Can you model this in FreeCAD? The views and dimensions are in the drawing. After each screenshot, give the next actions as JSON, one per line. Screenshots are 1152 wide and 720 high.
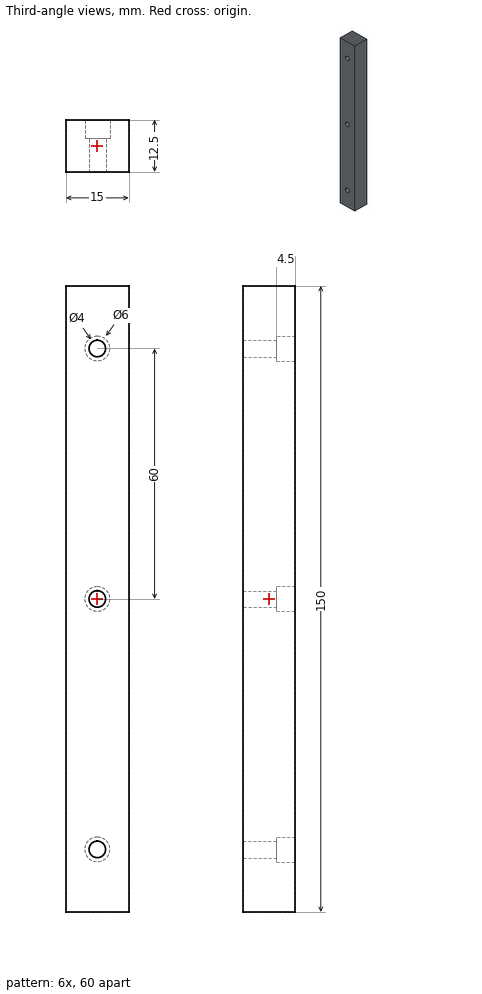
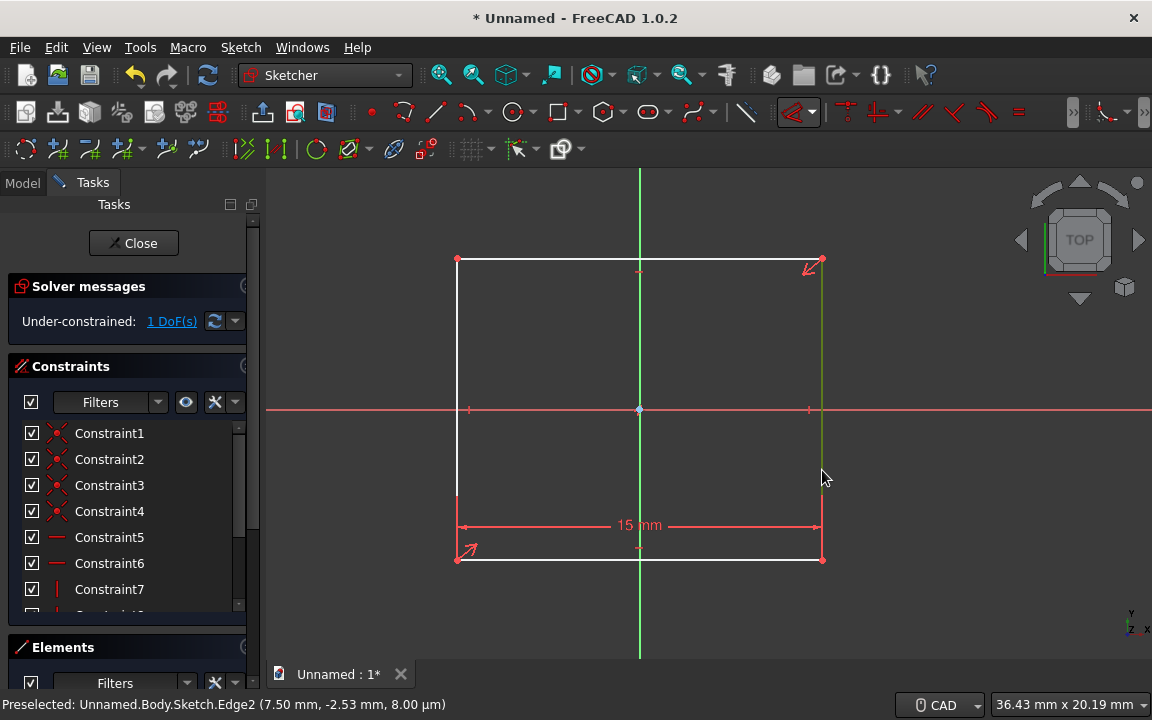
{"action": "key", "text": "i"}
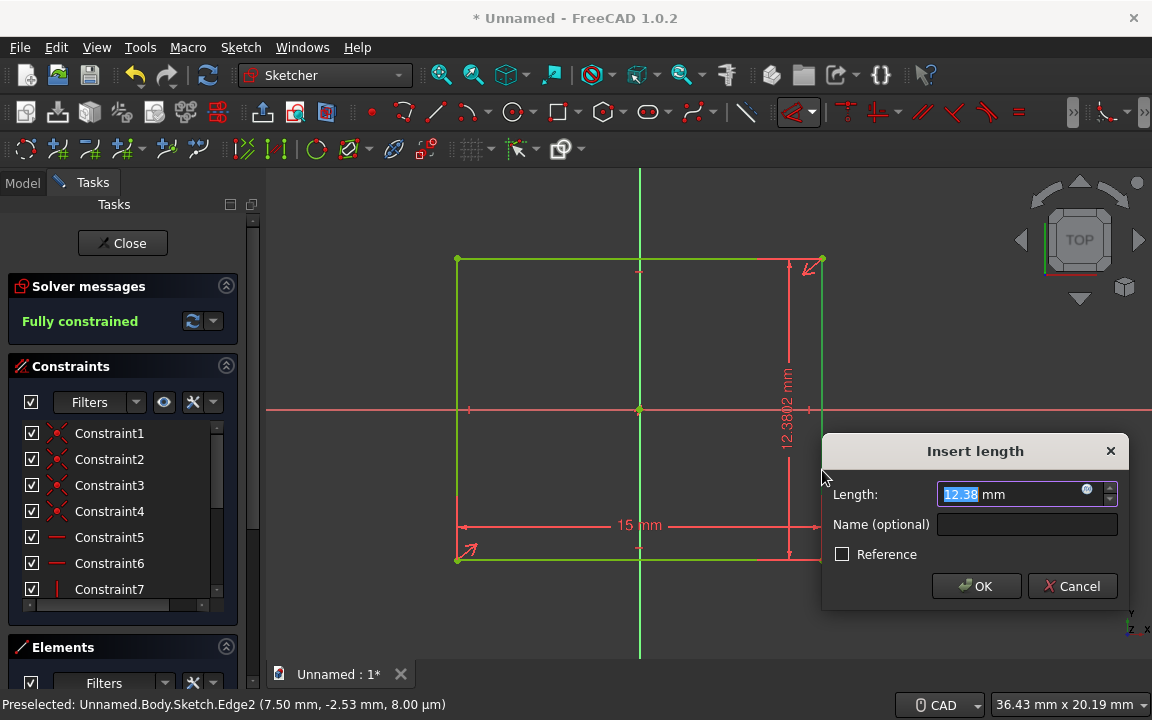
{"action": "type", "text": "12.5"}
{"action": "key", "text": "Return"}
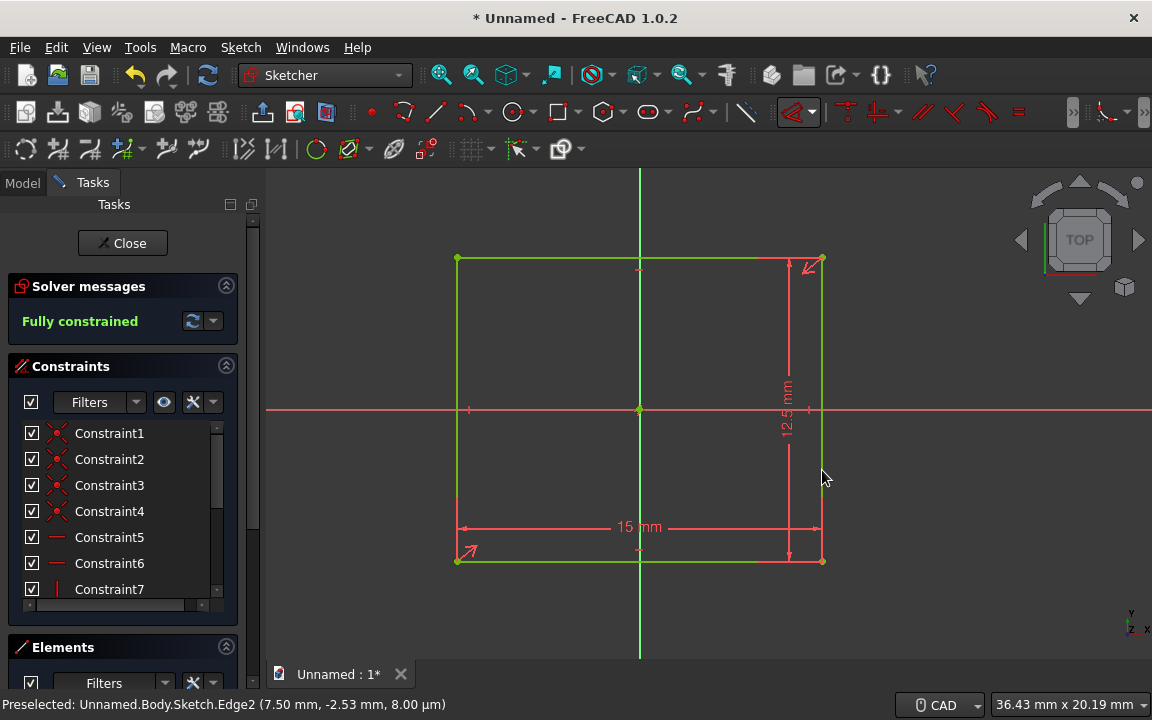
{"action": "left_click", "coordinate": [123, 243]}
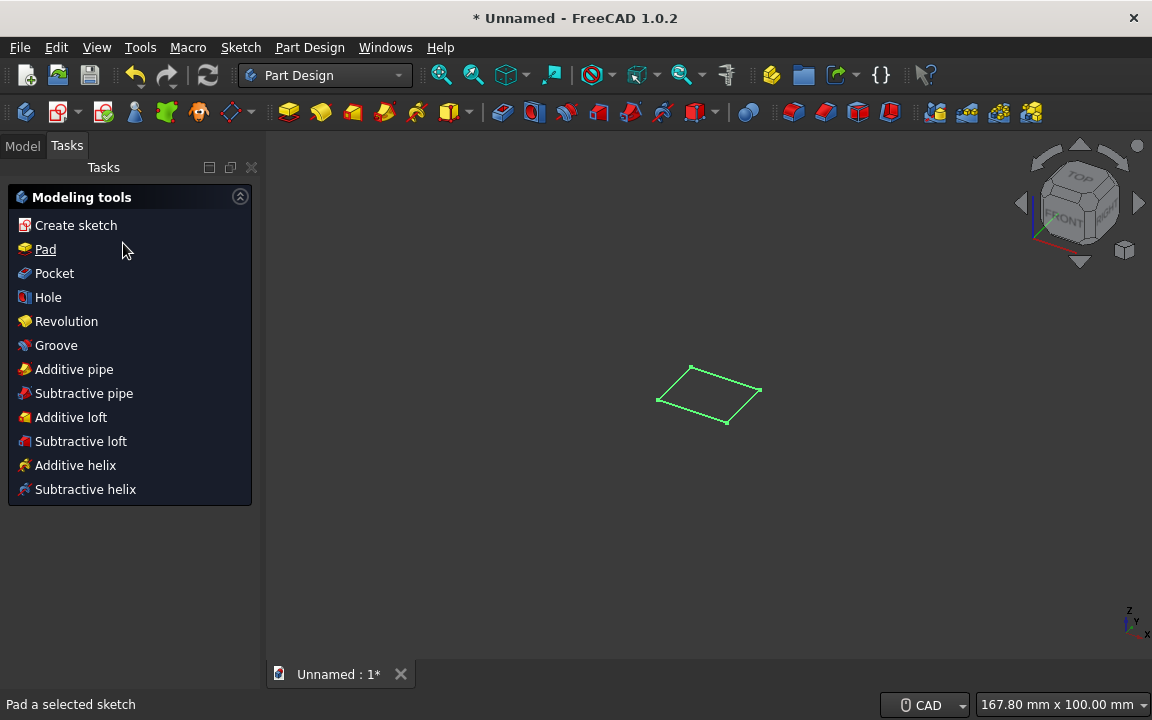
{"action": "left_click", "coordinate": [290, 112]}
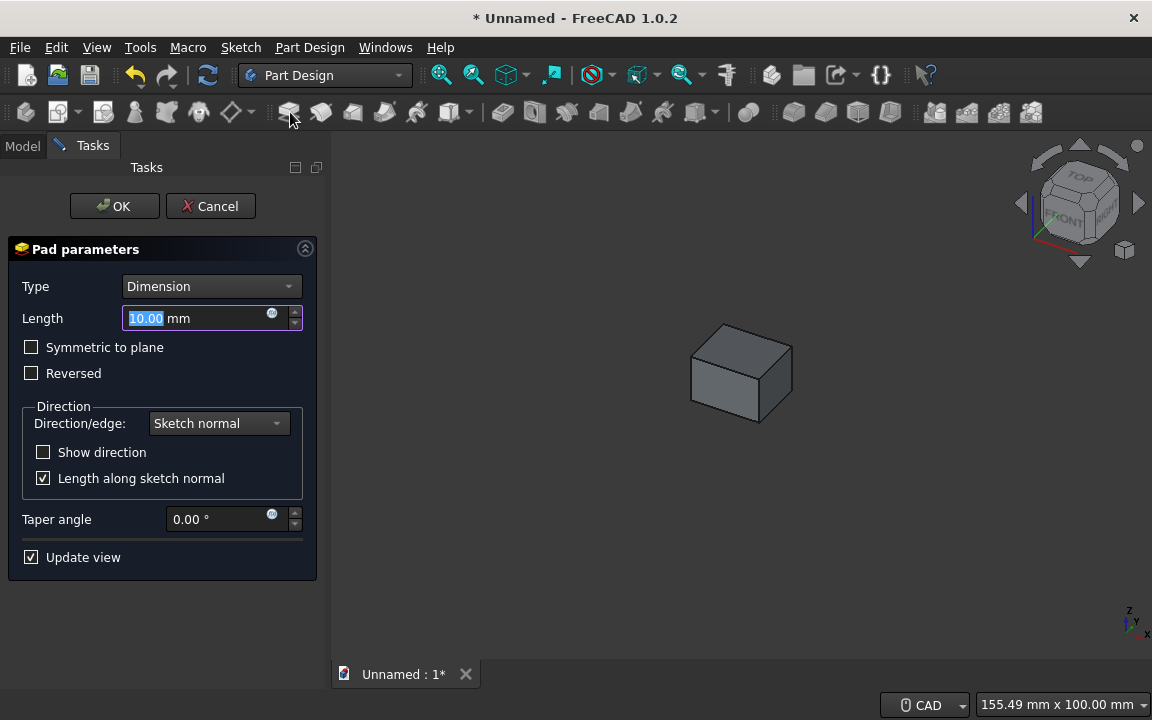
{"action": "type", "text": "150"}
{"action": "key", "text": "Tab"}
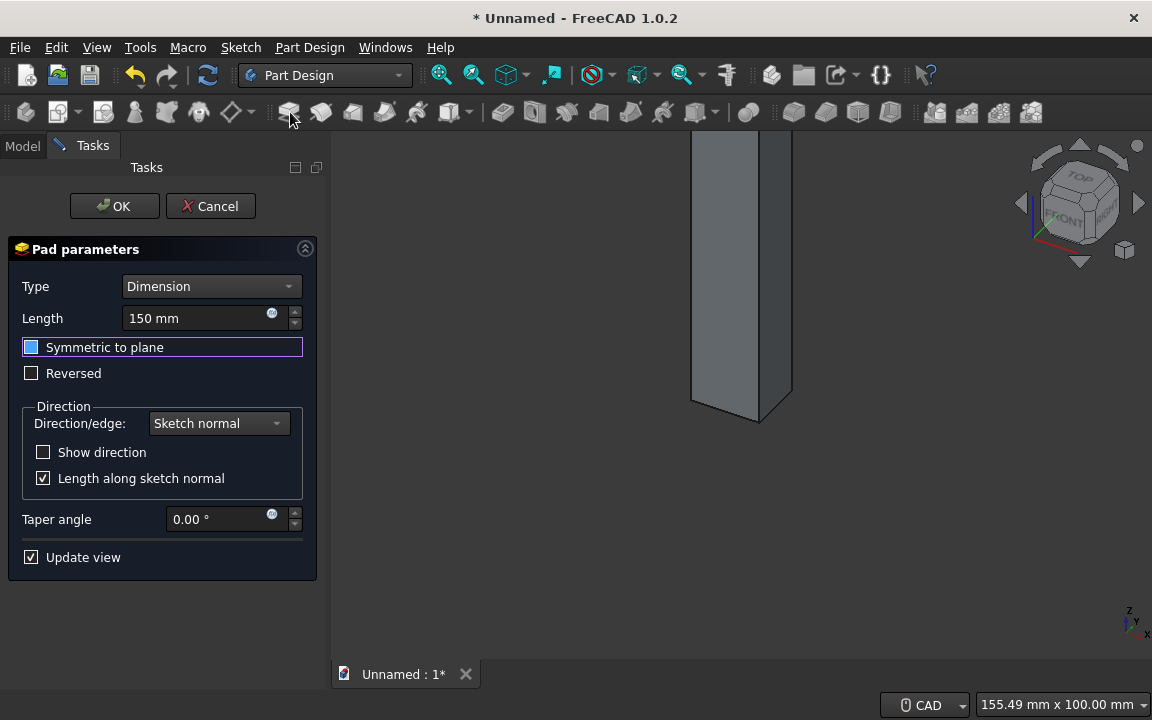
{"action": "left_click", "coordinate": [30, 347]}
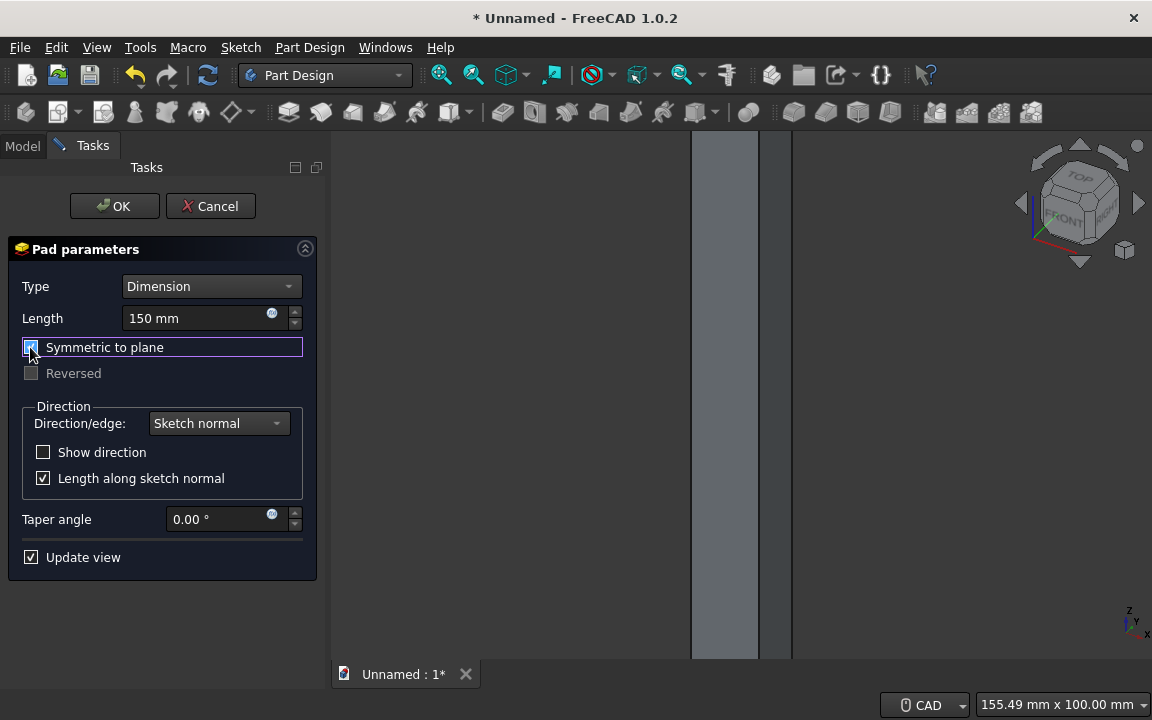
{"action": "left_click", "coordinate": [115, 206]}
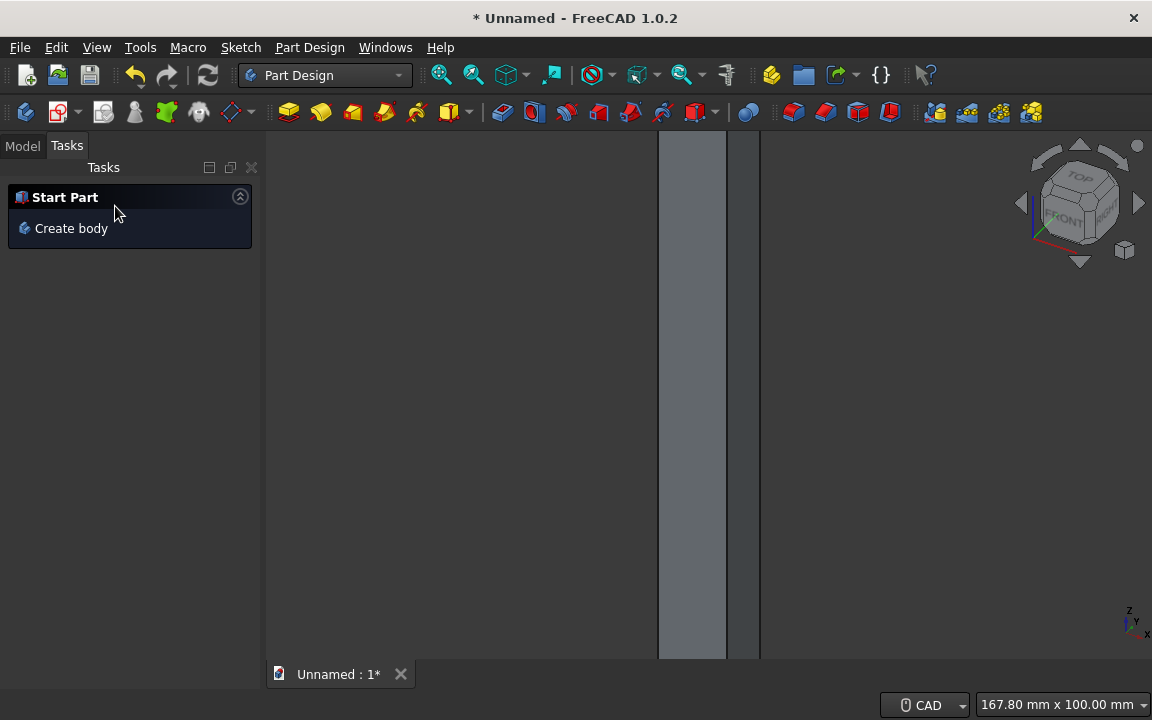
{"action": "key", "text": "v f"}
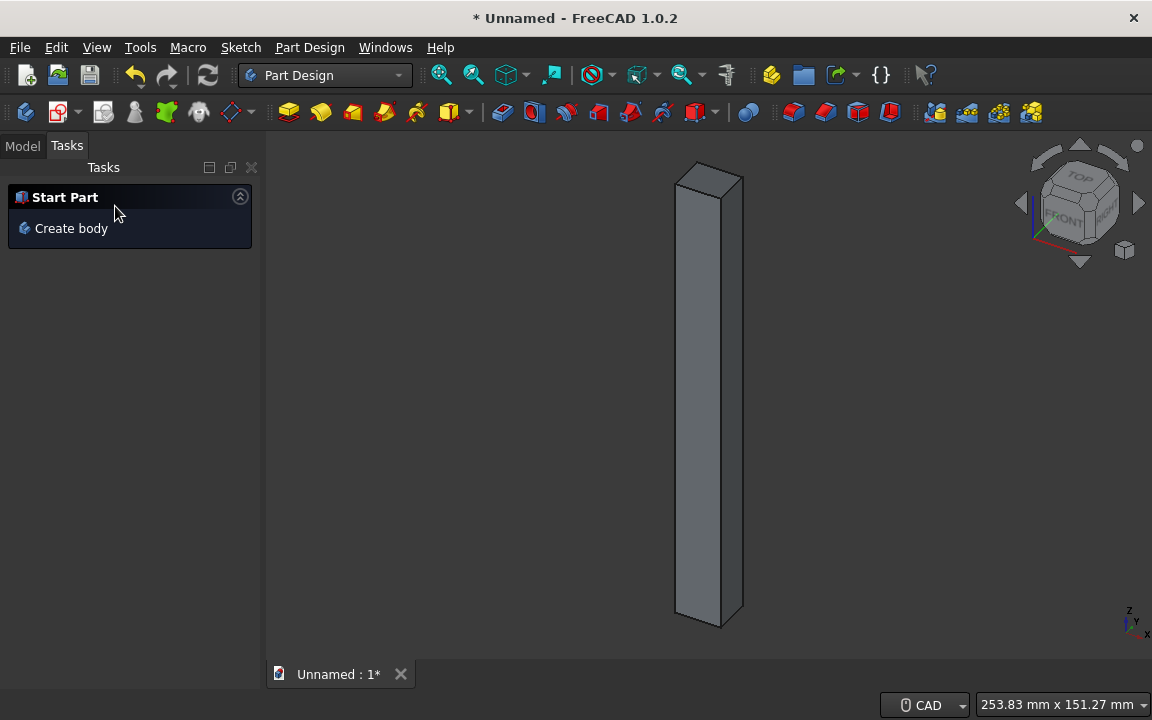
{"action": "key", "text": "4"}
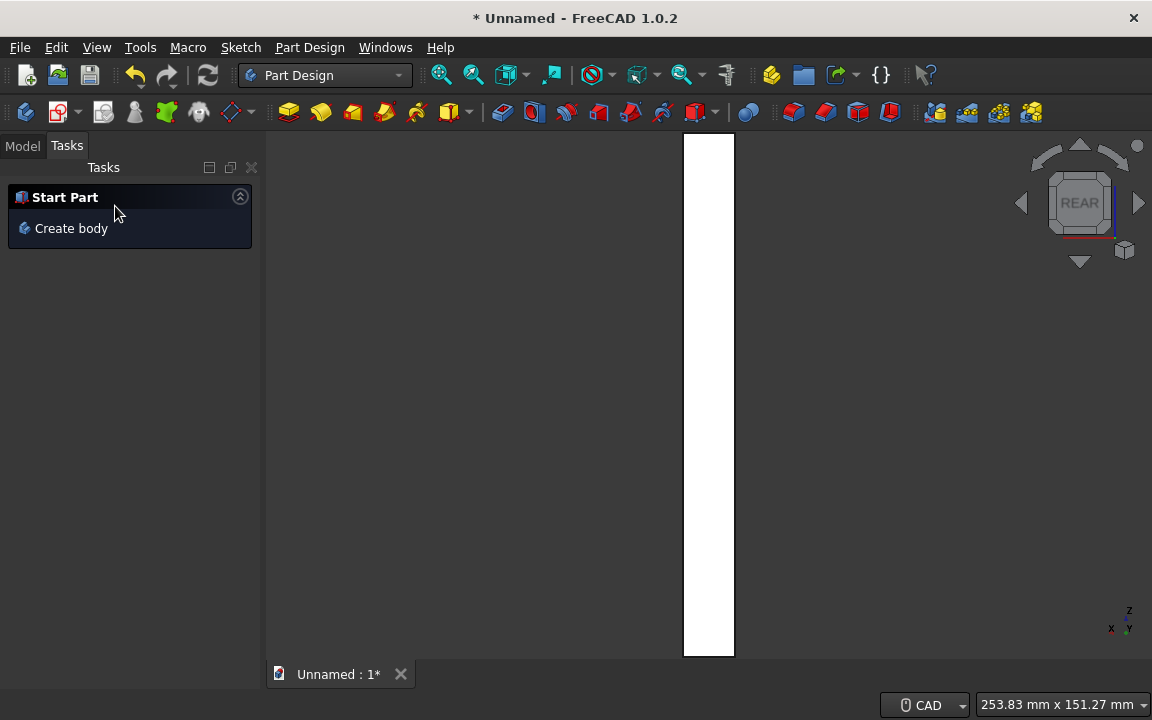
{"action": "left_click", "coordinate": [709, 170]}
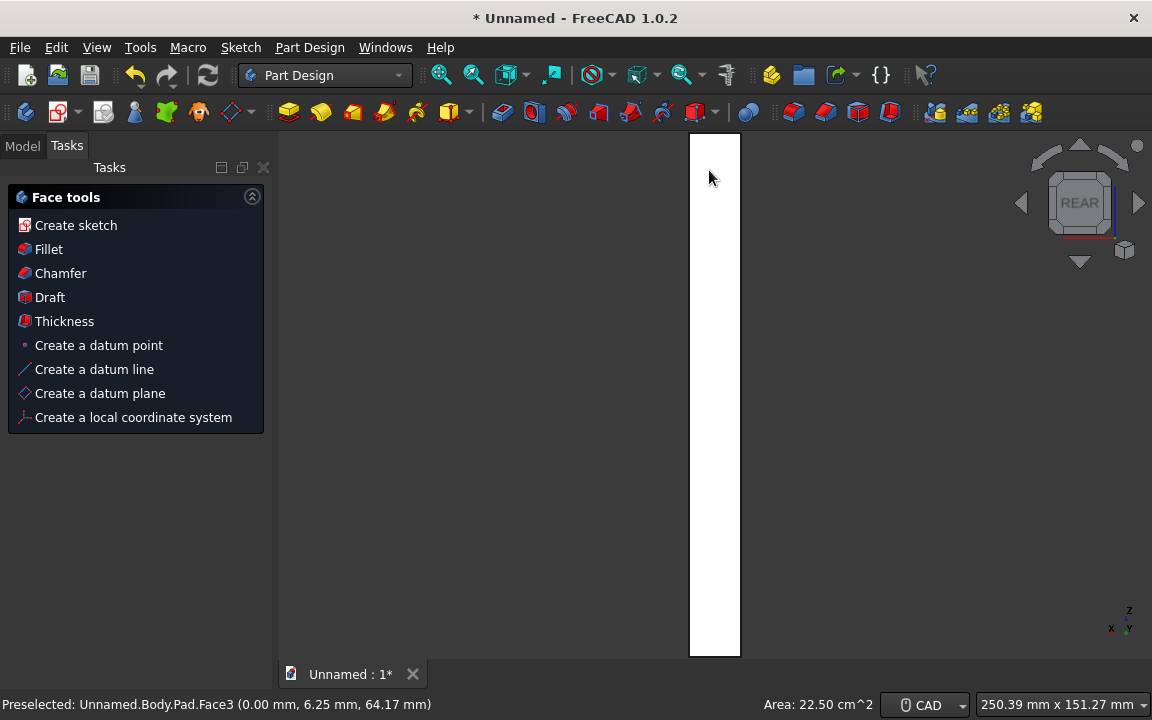
{"action": "left_click", "coordinate": [58, 112]}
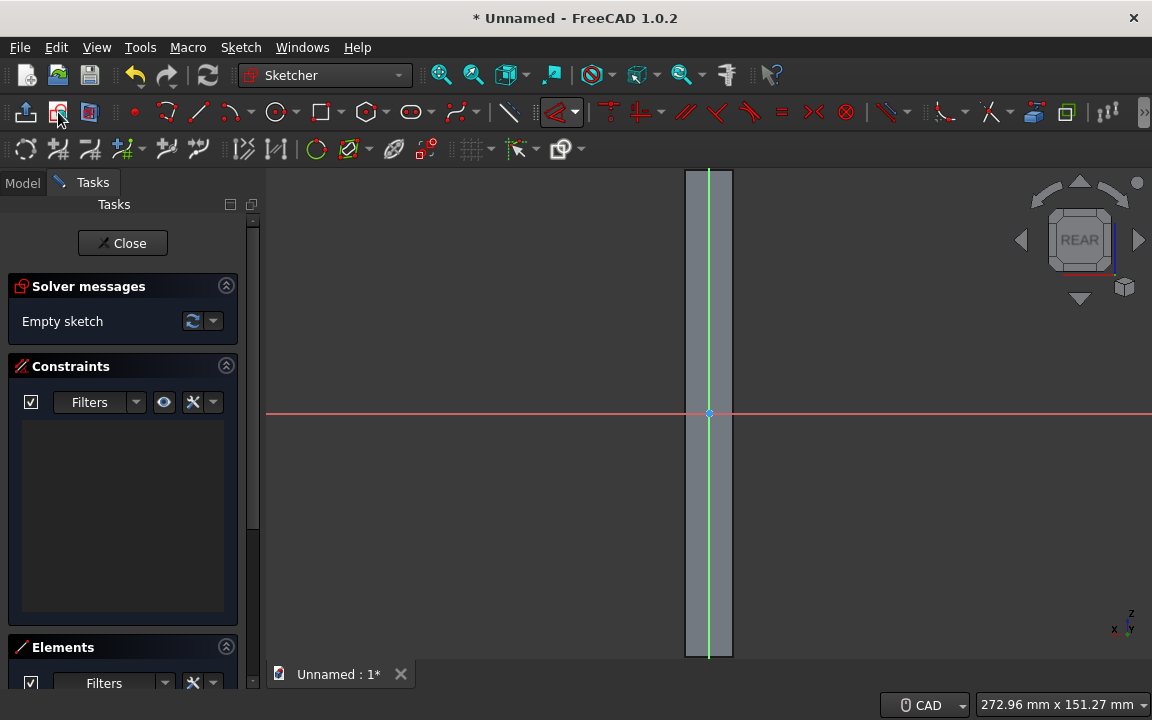
{"action": "scroll", "coordinate": [713, 206], "scroll_direction": "up", "scroll_amount": 14}